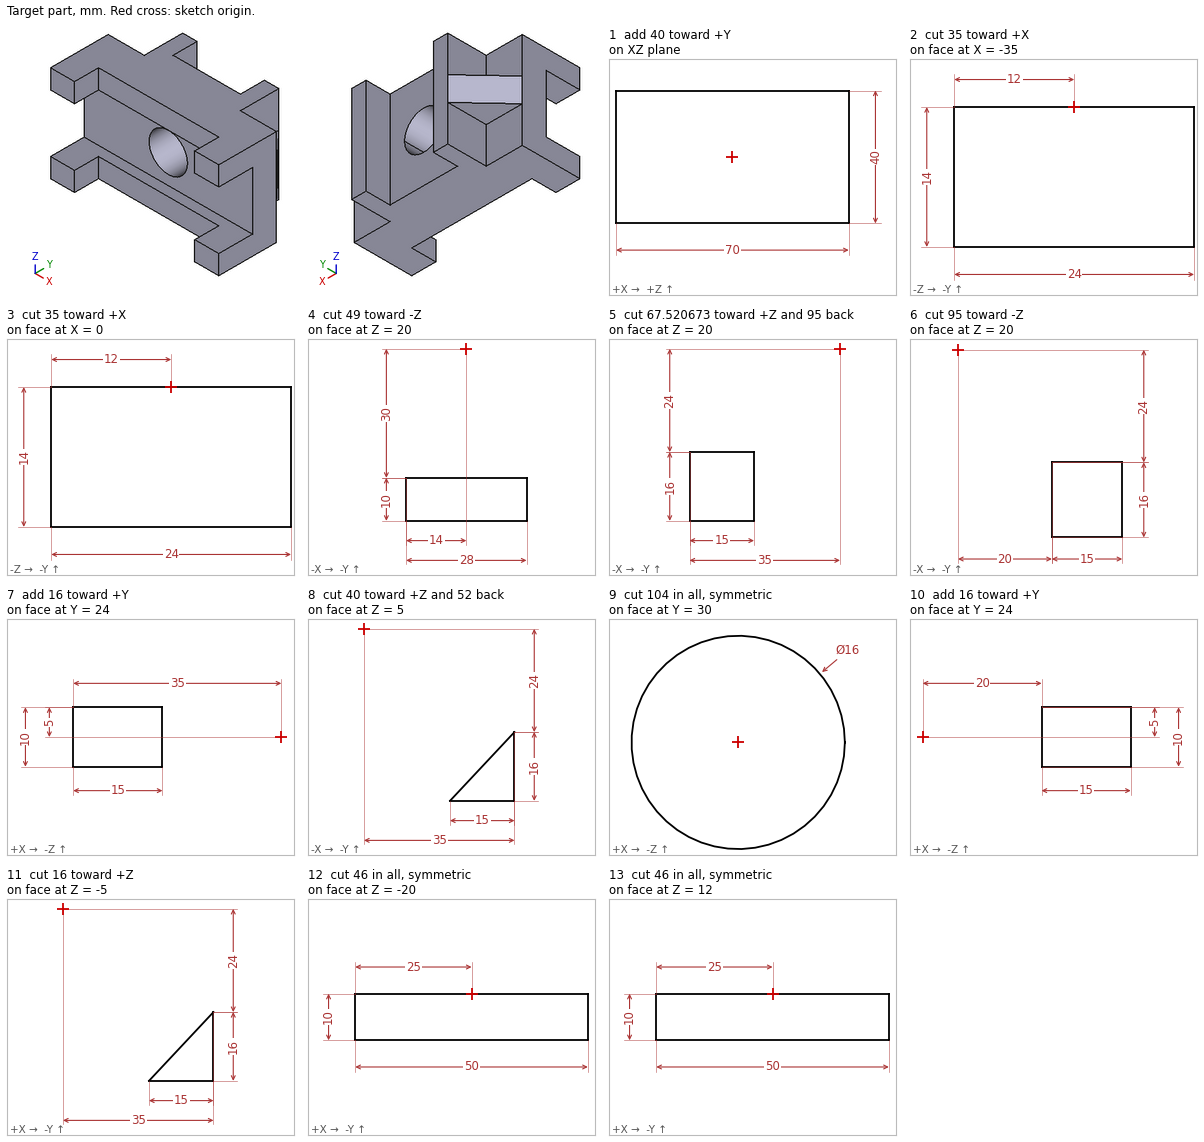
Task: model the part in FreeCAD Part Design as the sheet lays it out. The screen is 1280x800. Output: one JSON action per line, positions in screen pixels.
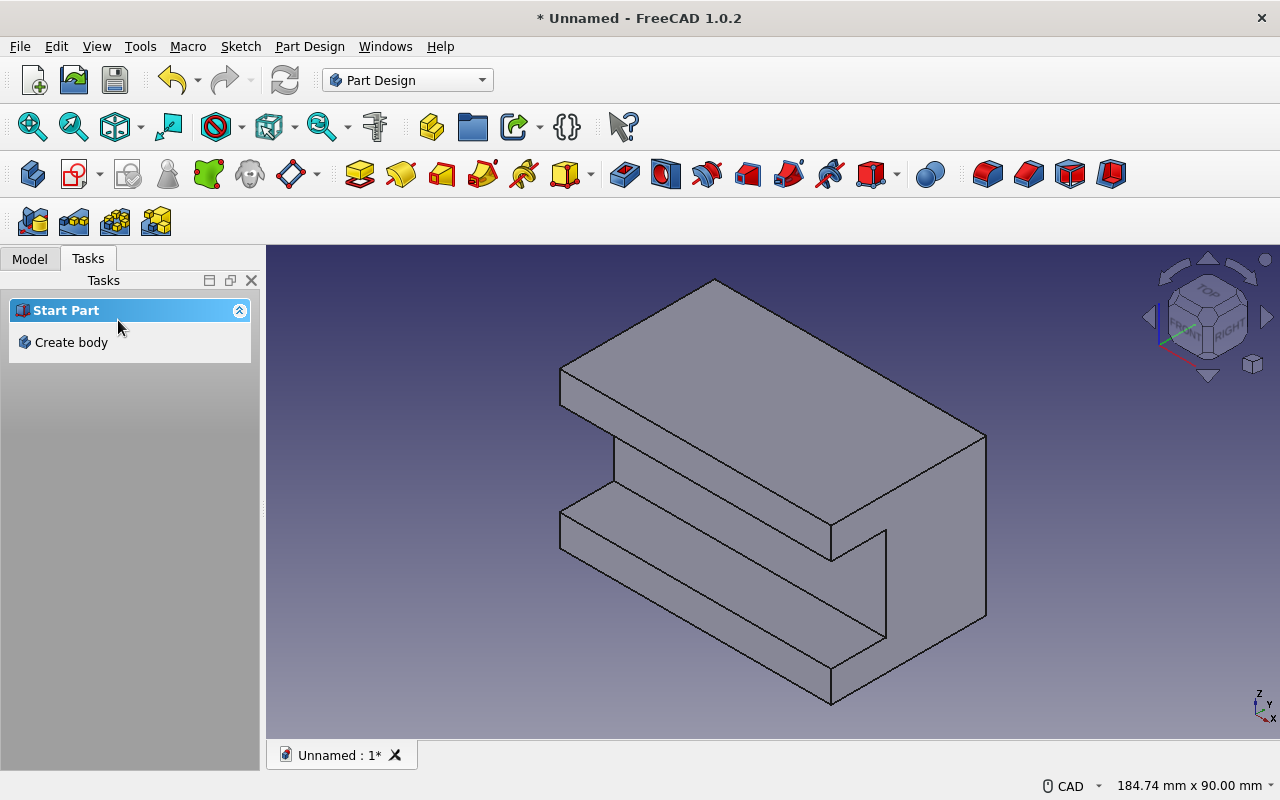
{"action": "left_click", "coordinate": [812, 424]}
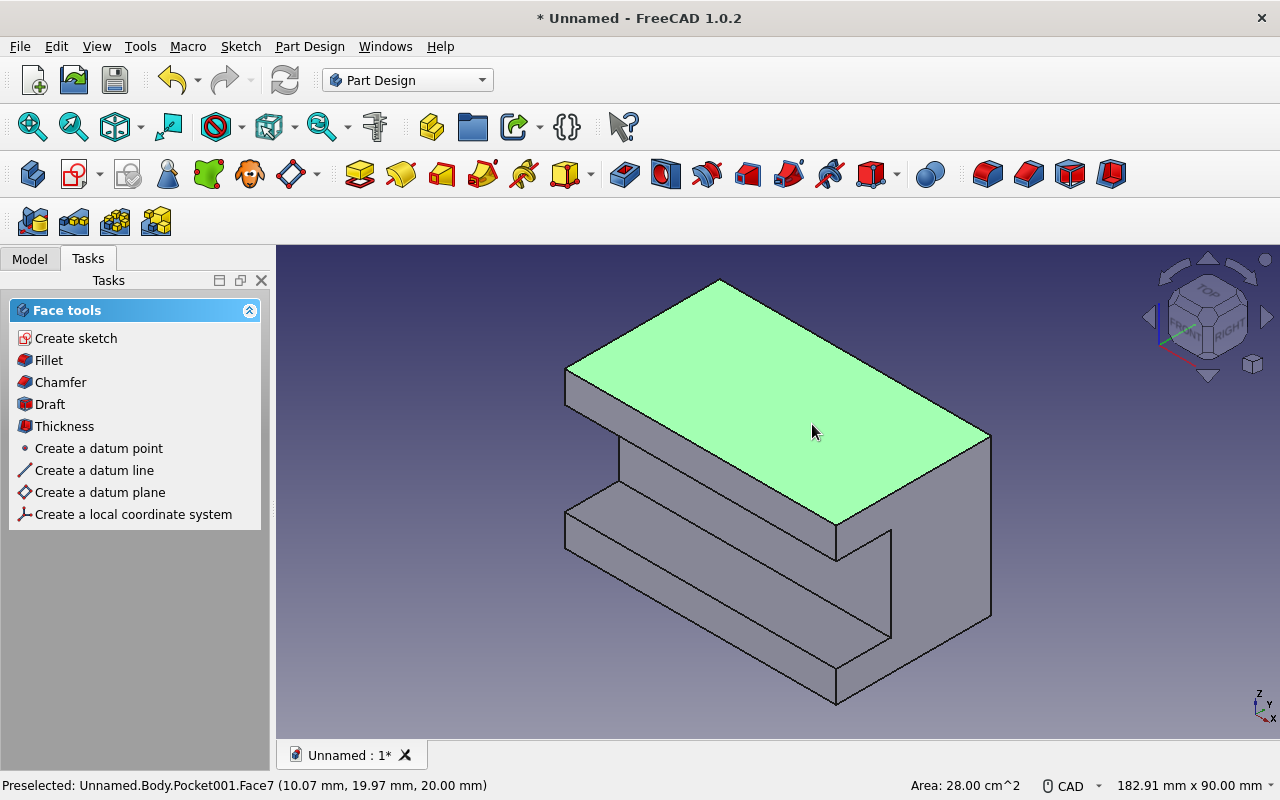
{"action": "left_click", "coordinate": [74, 174]}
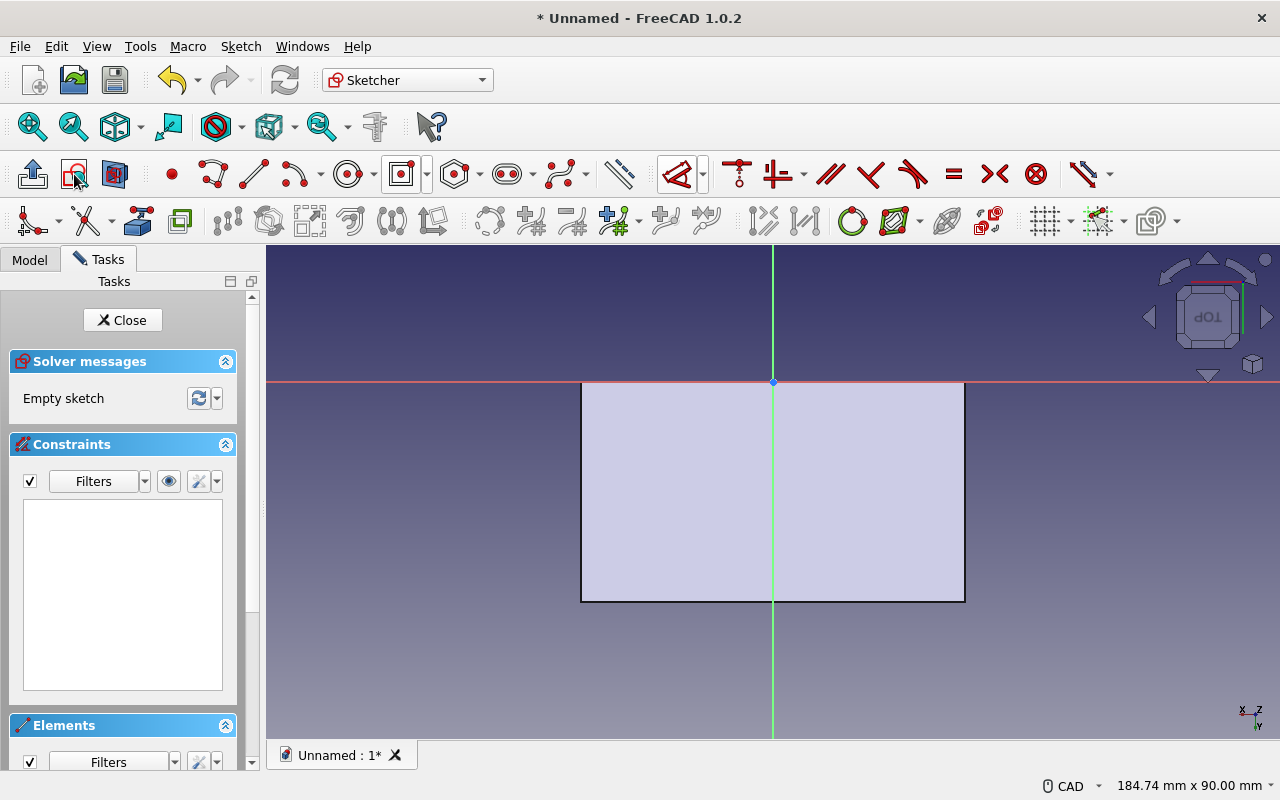
{"action": "scroll", "coordinate": [912, 492], "scroll_direction": "up", "scroll_amount": 2}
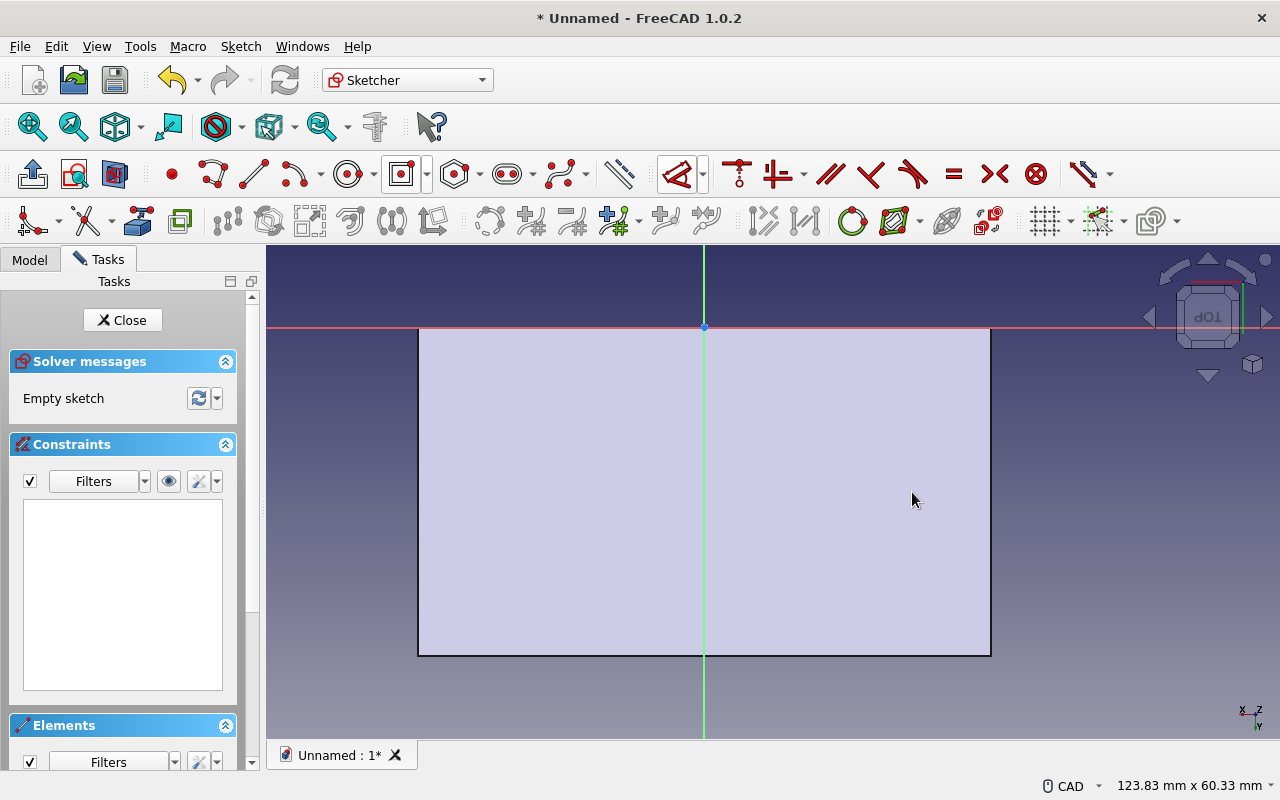
{"action": "key", "text": "g r"}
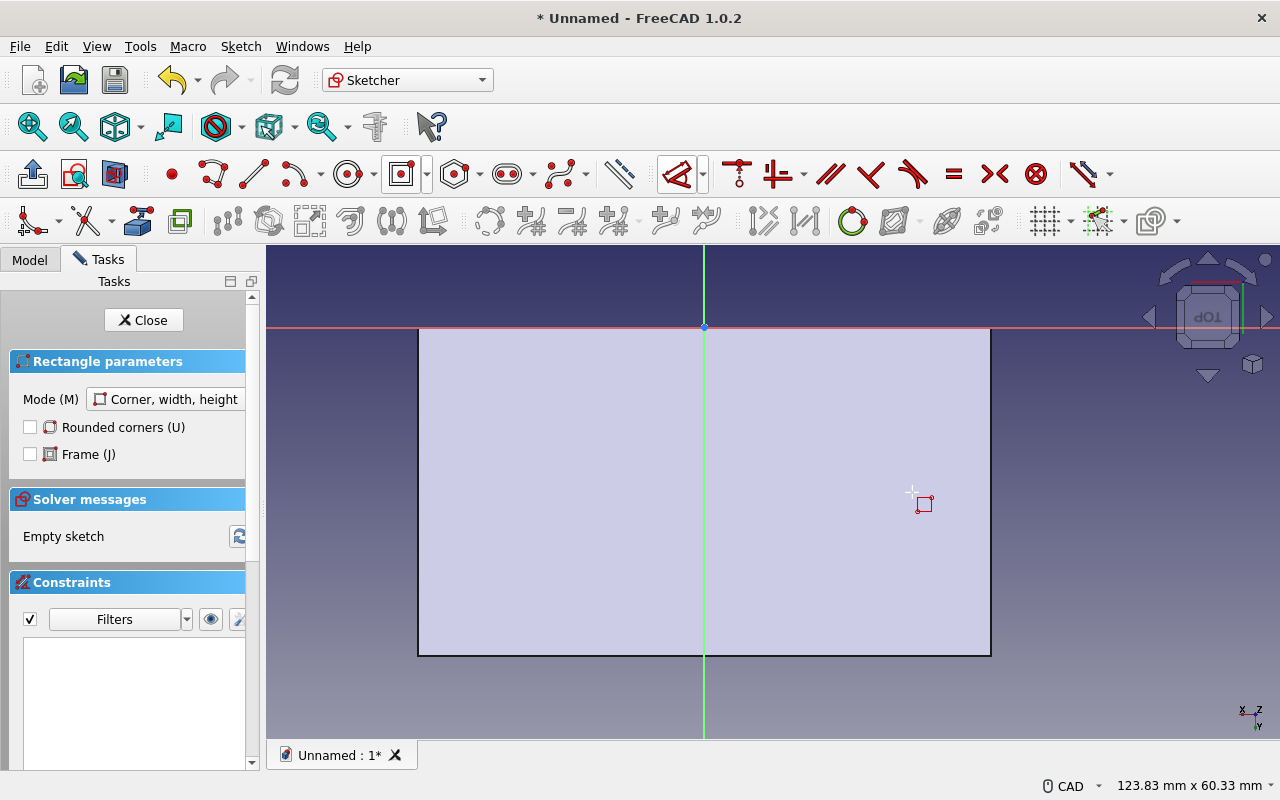
{"action": "left_click", "coordinate": [590, 574]}
{"action": "left_click", "coordinate": [819, 656]}
{"action": "key", "text": "Escape"}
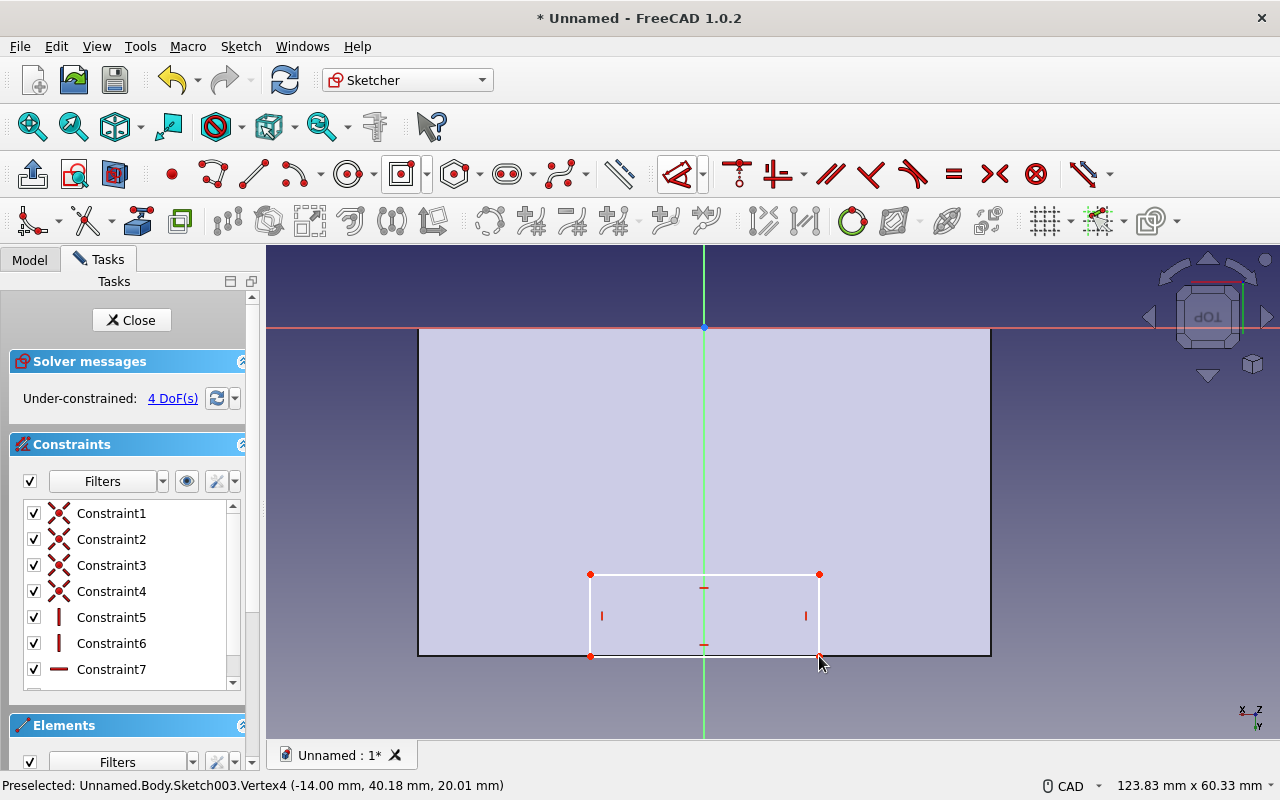
{"action": "left_click", "coordinate": [590, 600]}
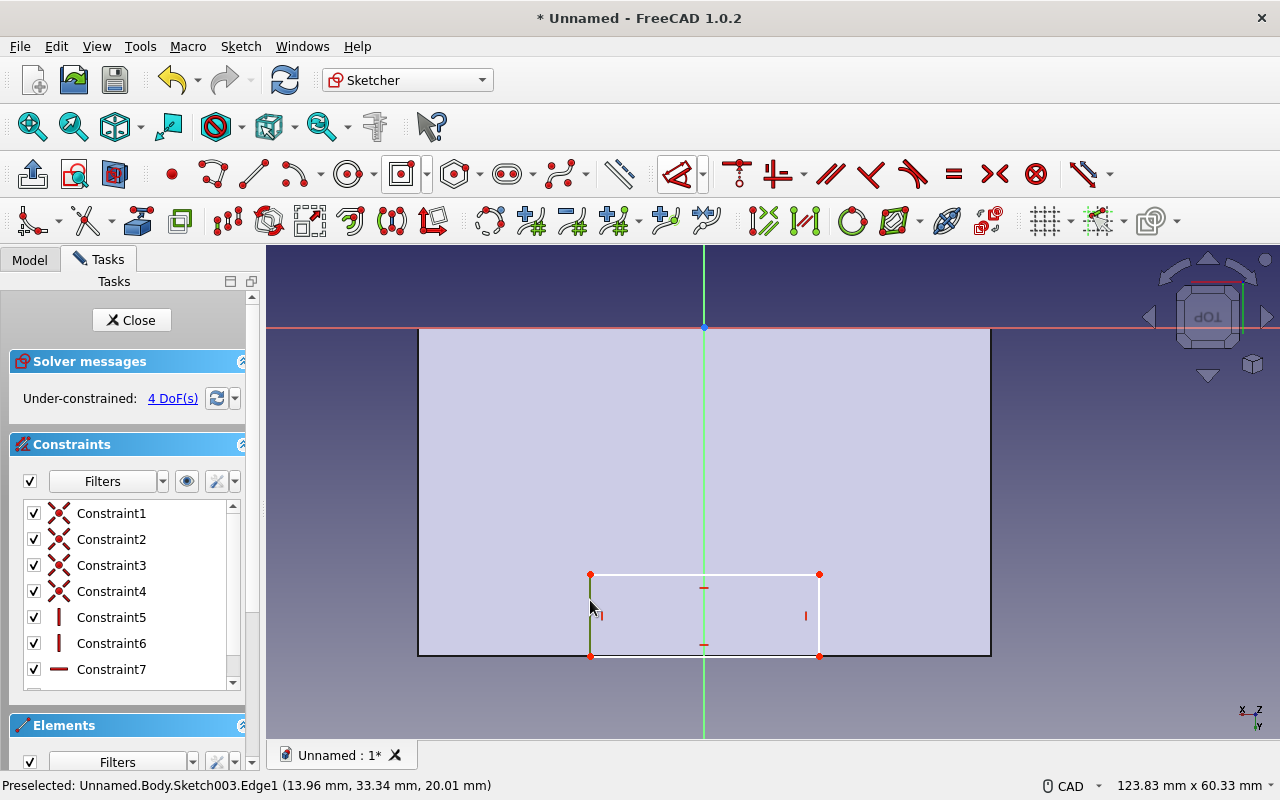
{"action": "key", "text": "i"}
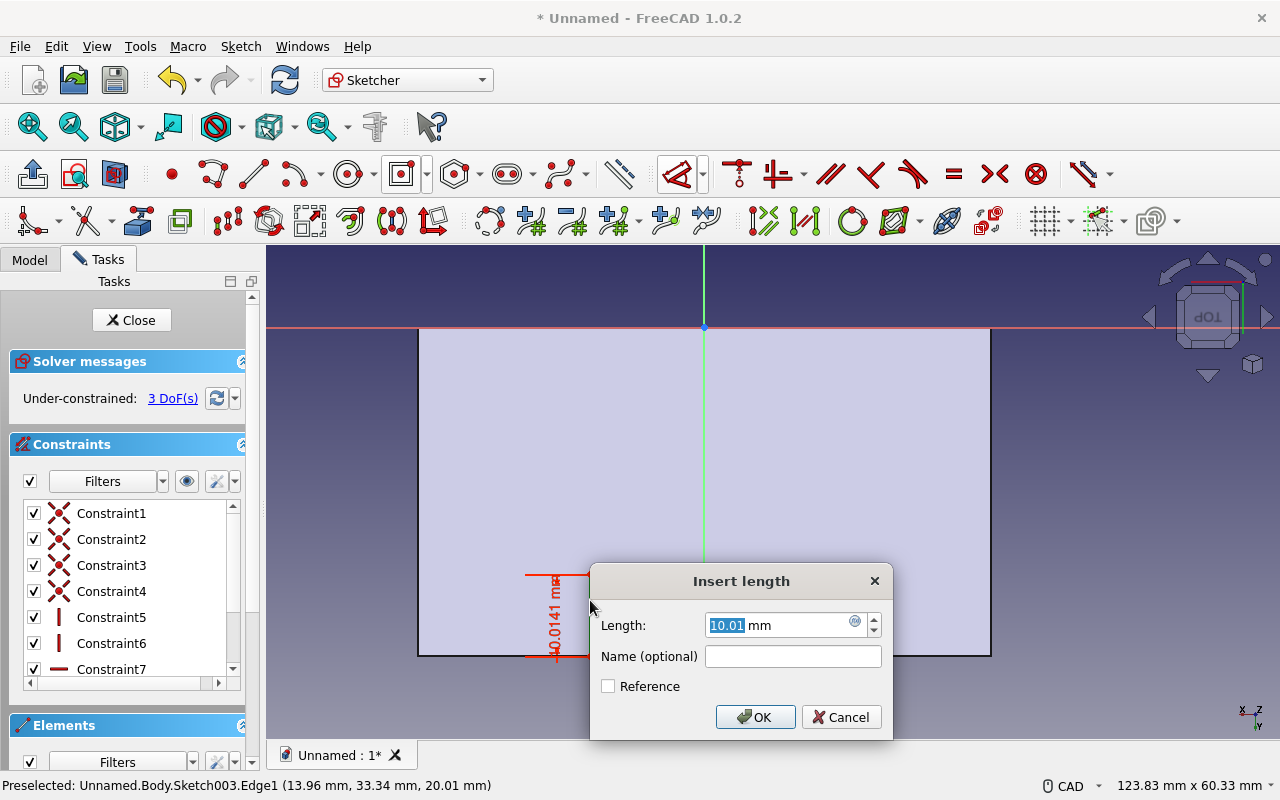
{"action": "type", "text": "10"}
{"action": "key", "text": "Return"}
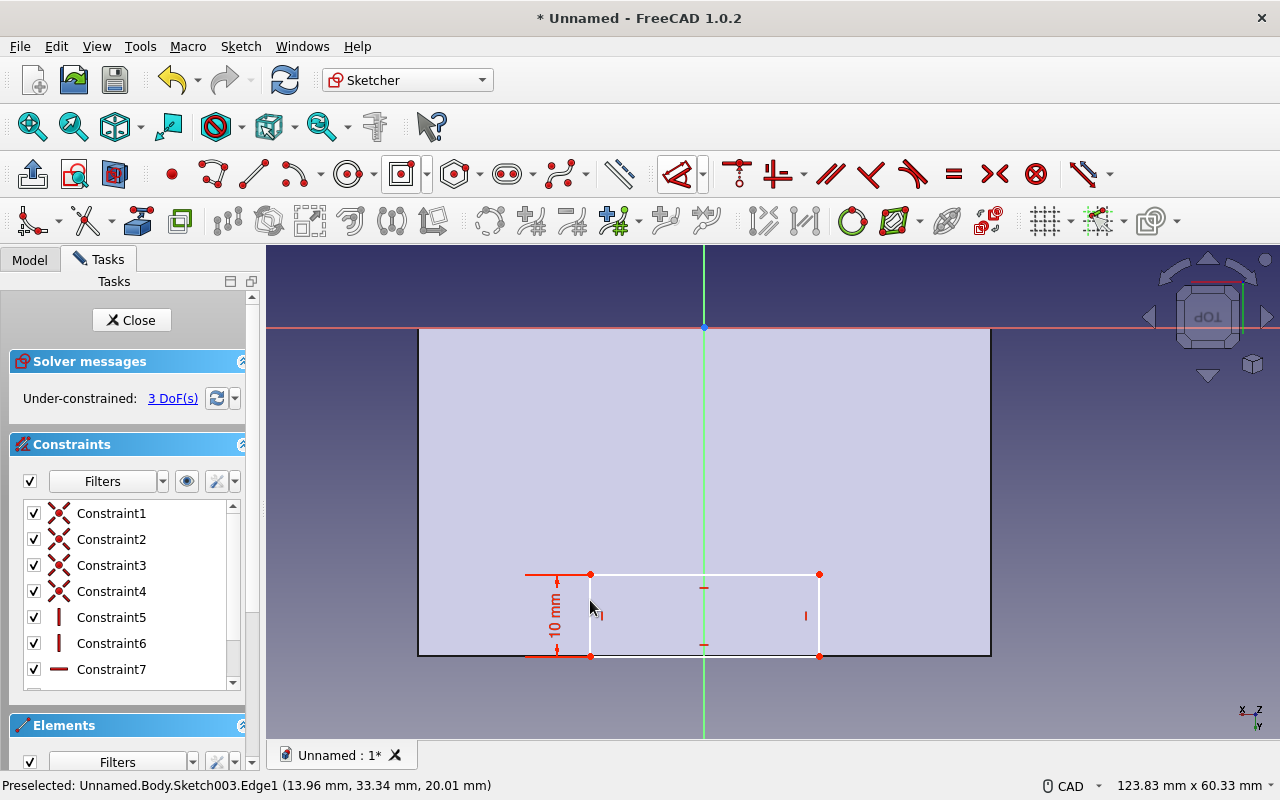
{"action": "left_click", "coordinate": [659, 657]}